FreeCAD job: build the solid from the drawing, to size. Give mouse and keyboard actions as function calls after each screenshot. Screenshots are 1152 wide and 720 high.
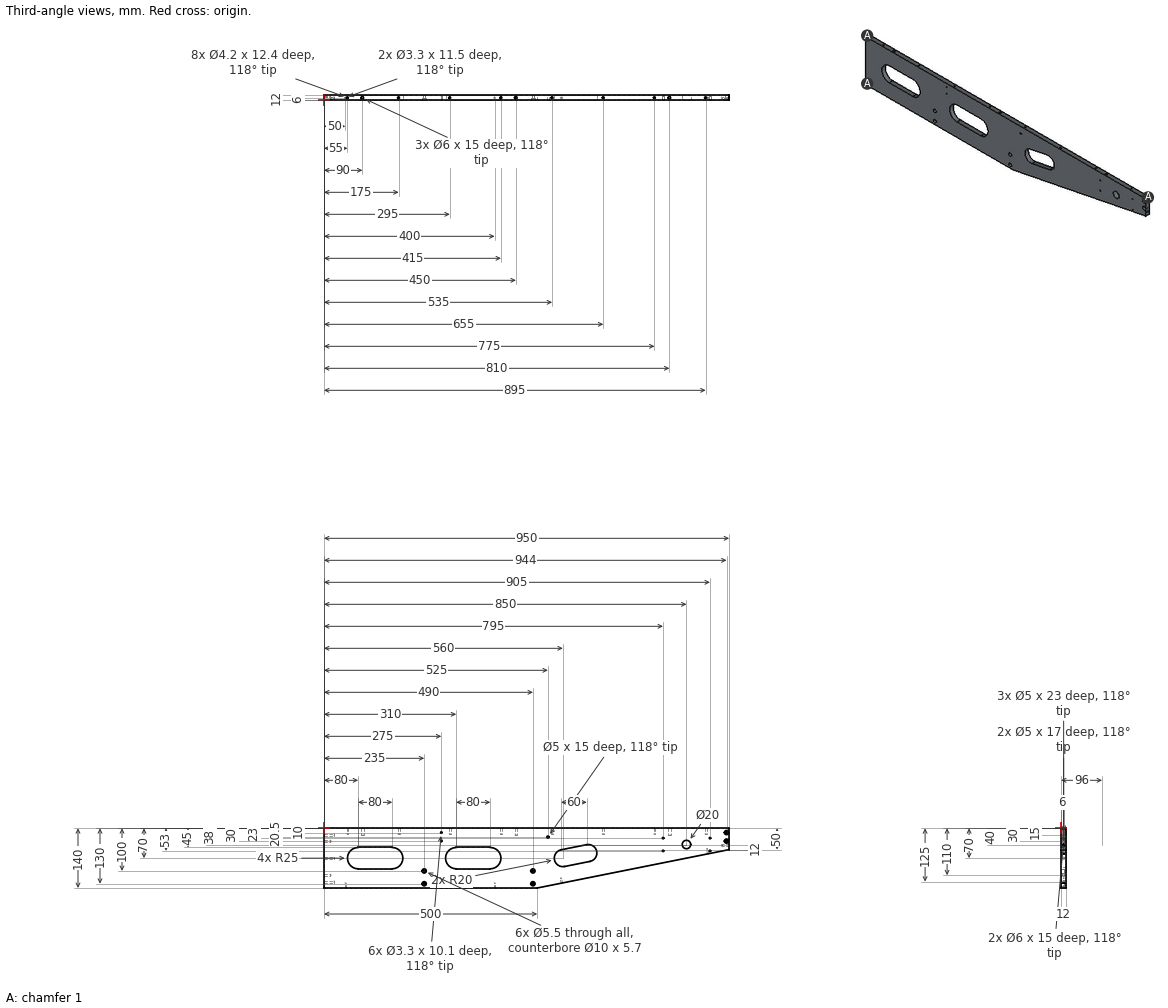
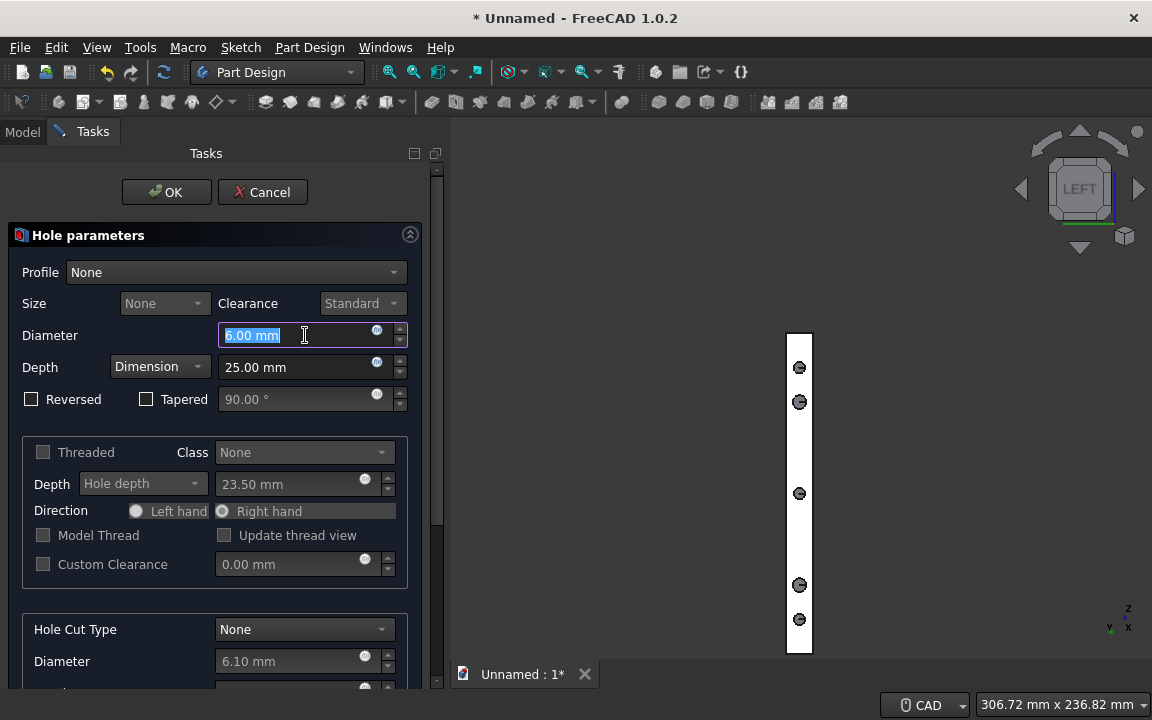
text(4.2)
key(Tab)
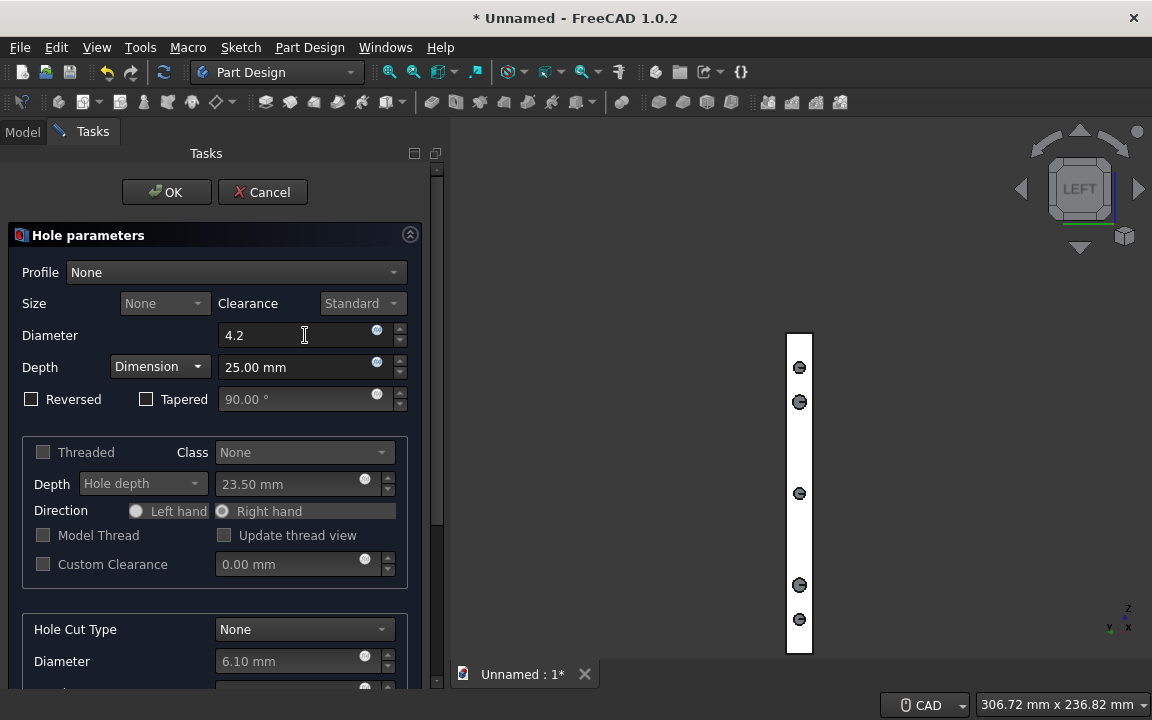
triple_click(305, 367)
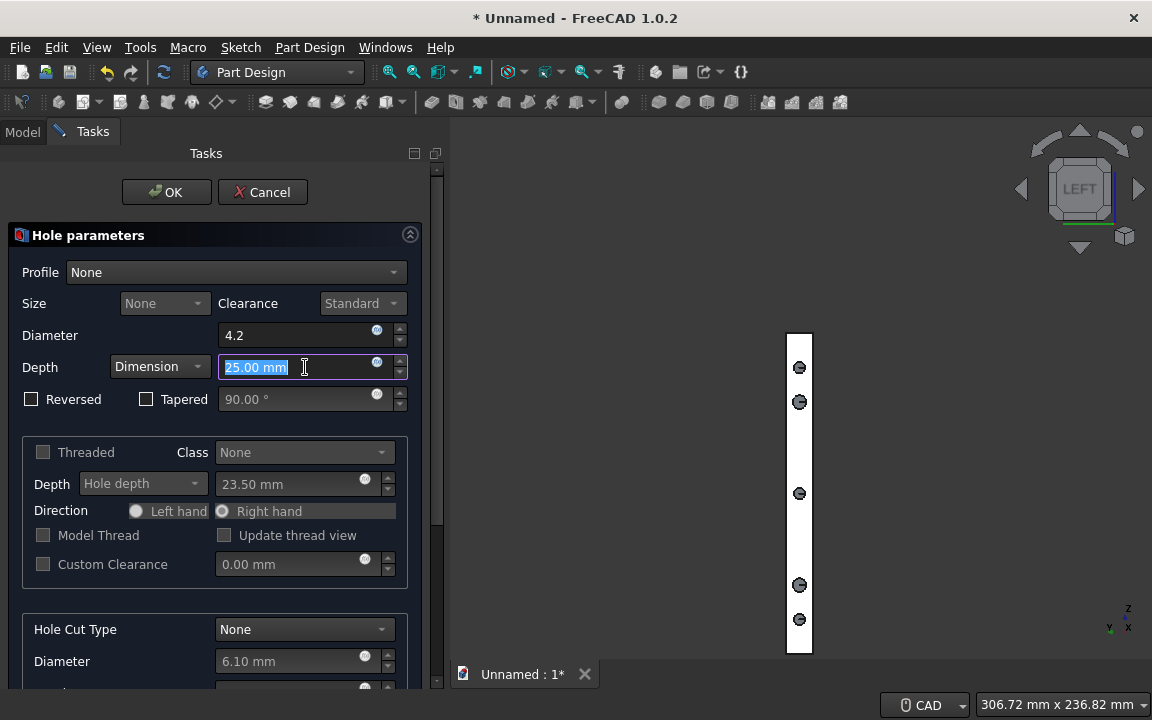
text(12.4)
key(Tab)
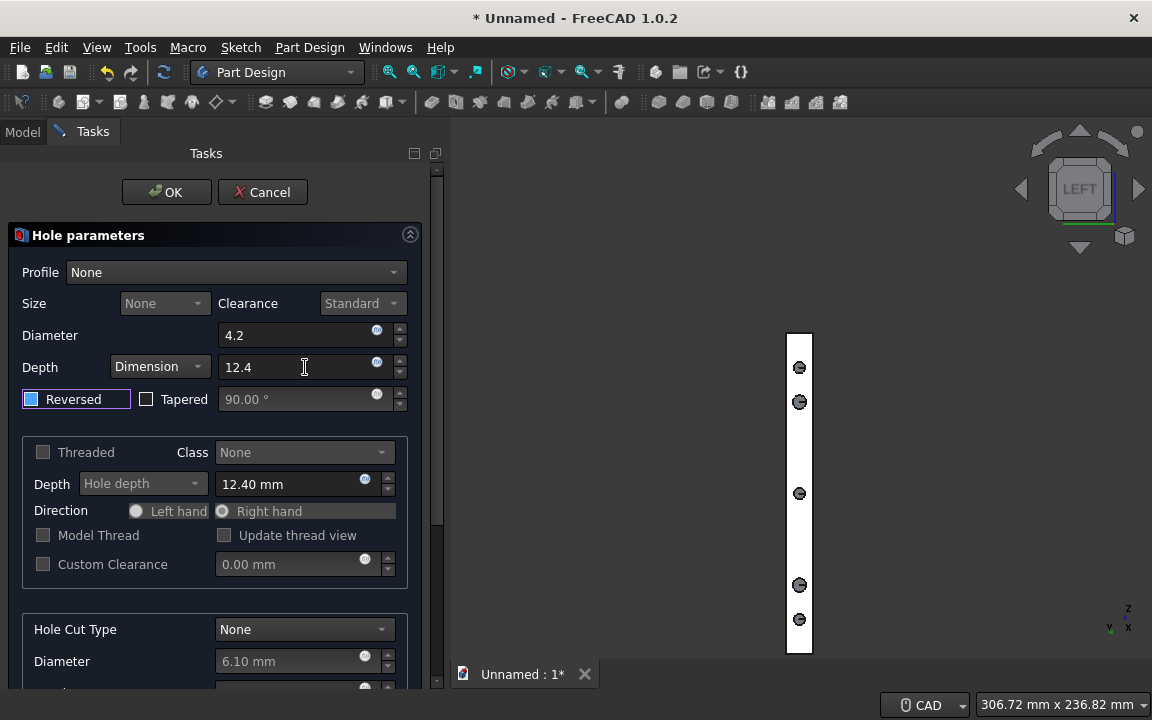
click(167, 192)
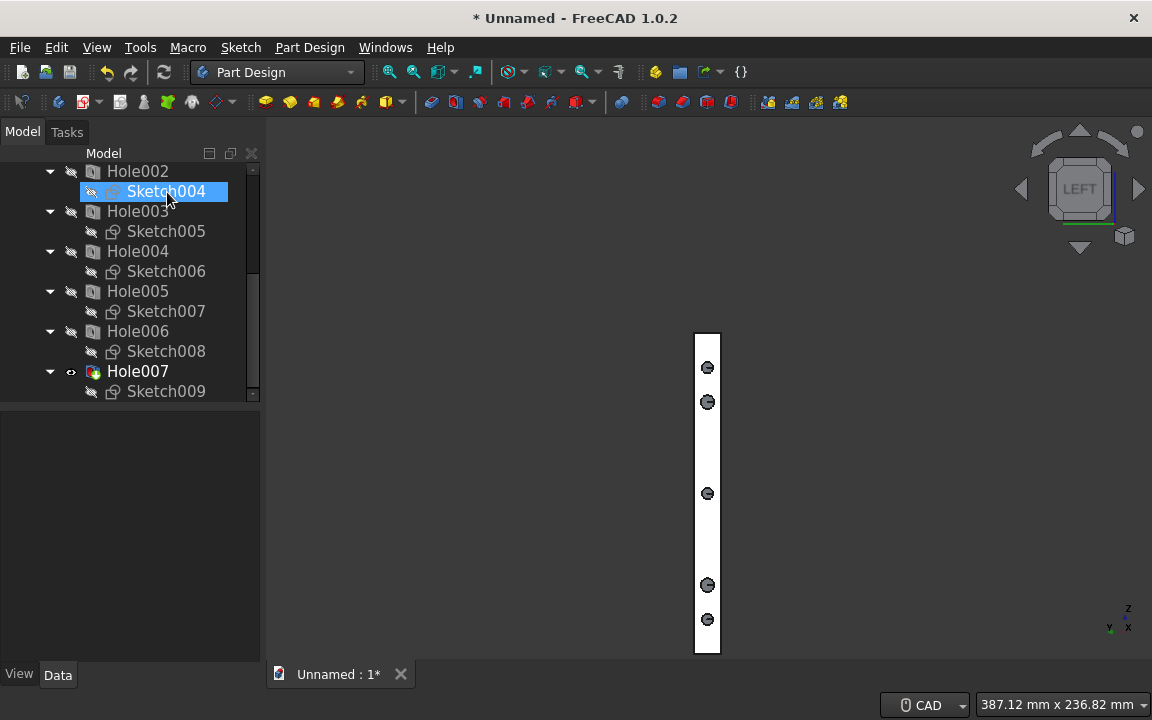
key(0)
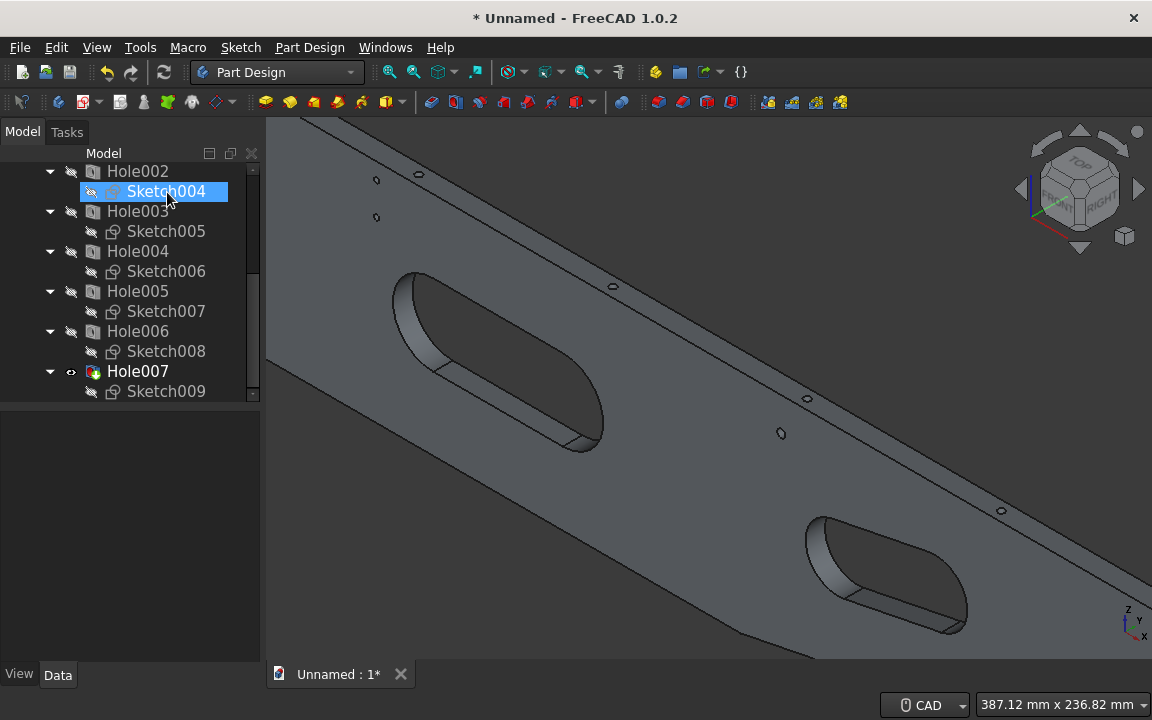
key(v)
key(f)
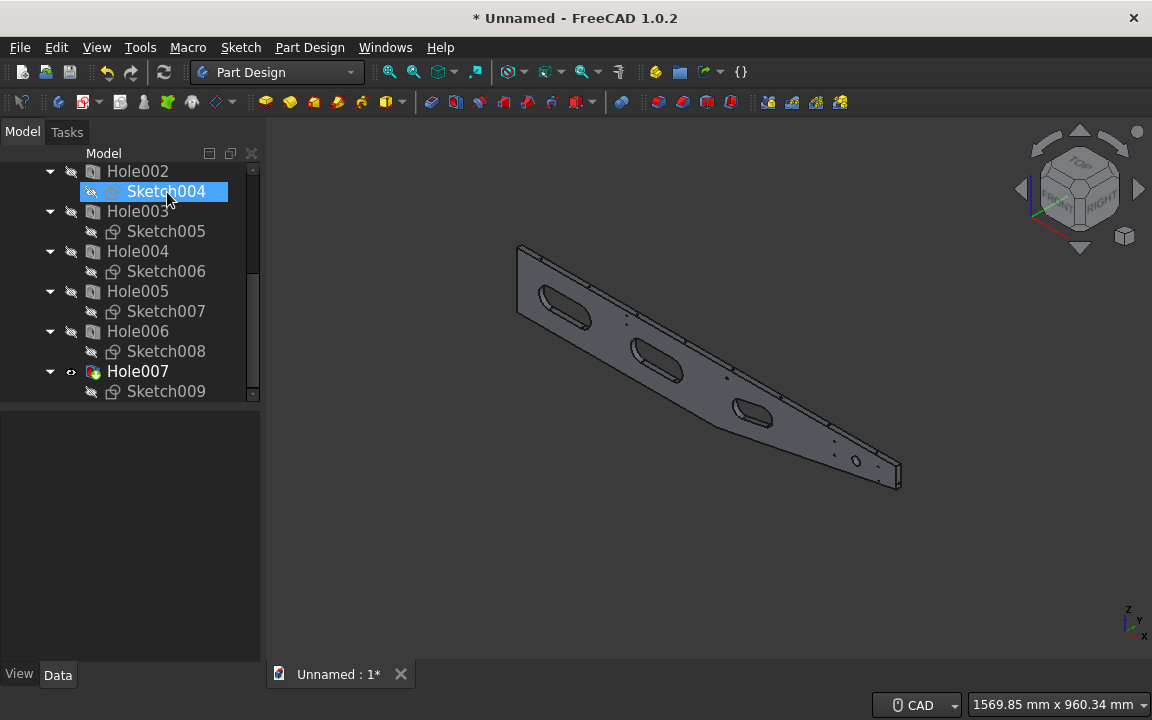
scroll(871, 449, up, 7)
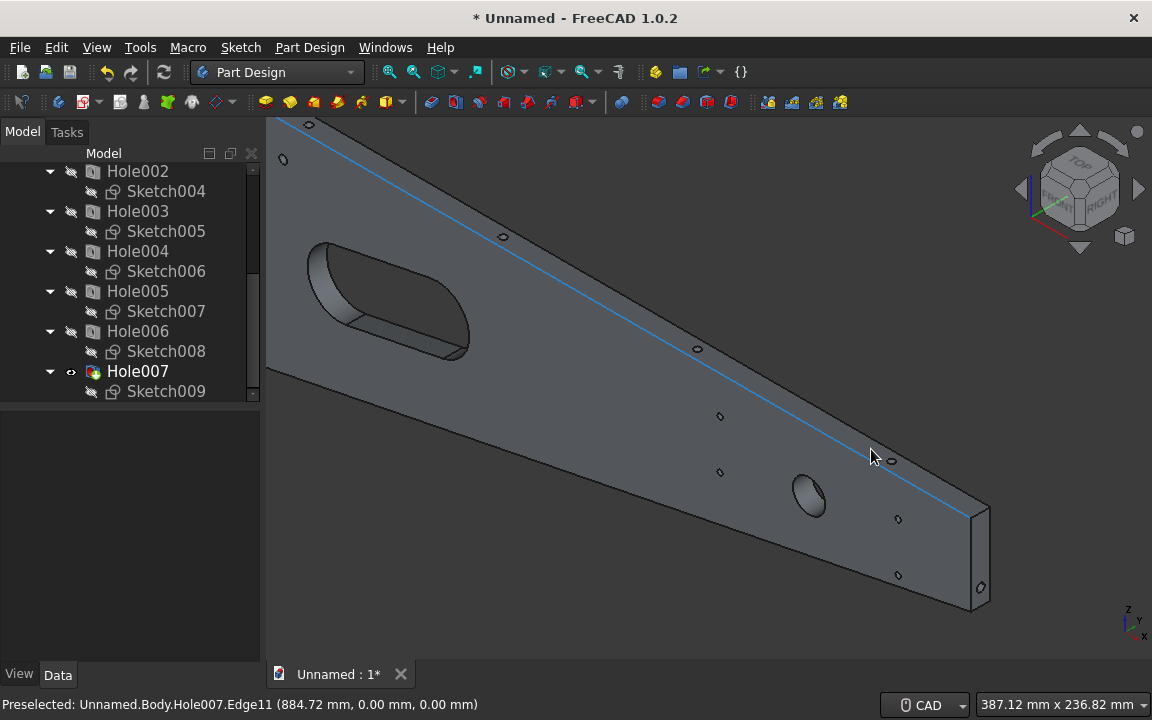
click(871, 448)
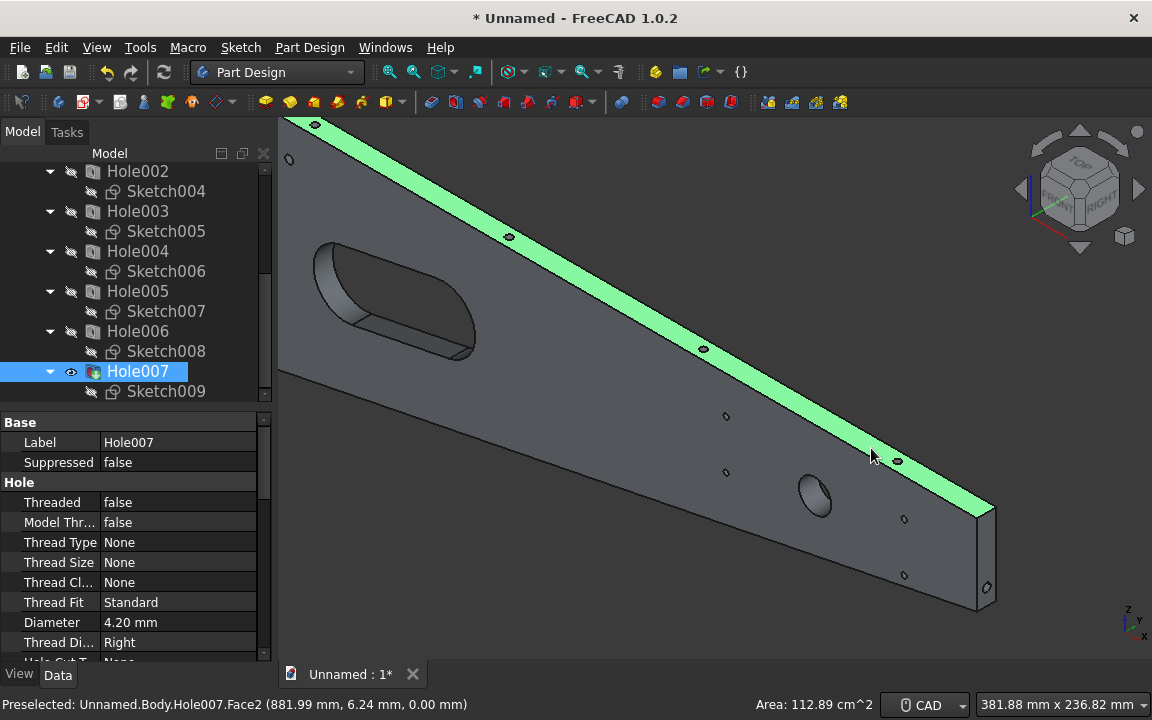
click(84, 102)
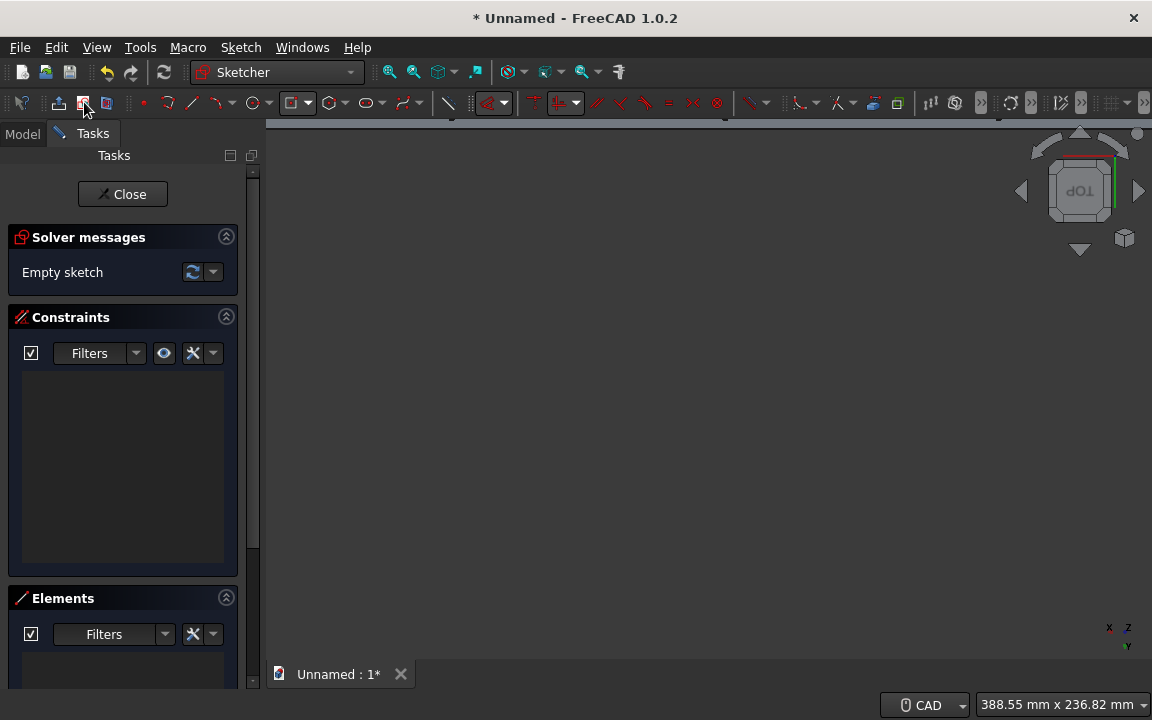
scroll(427, 480, down, 7)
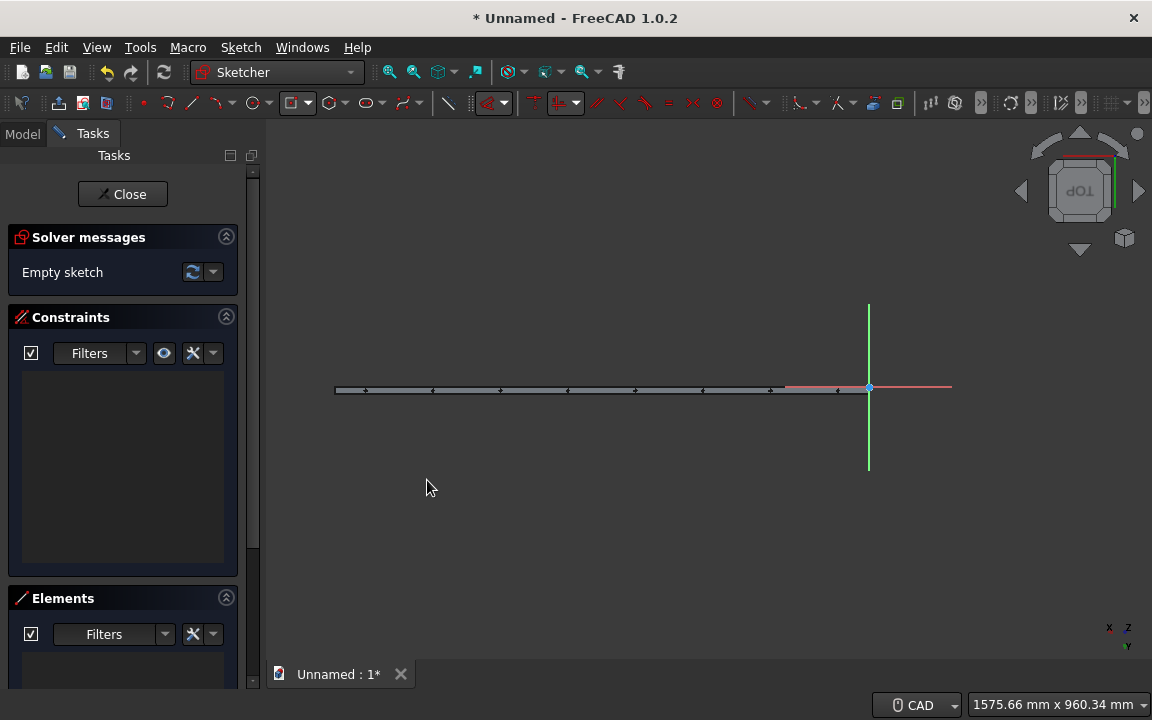
click(254, 104)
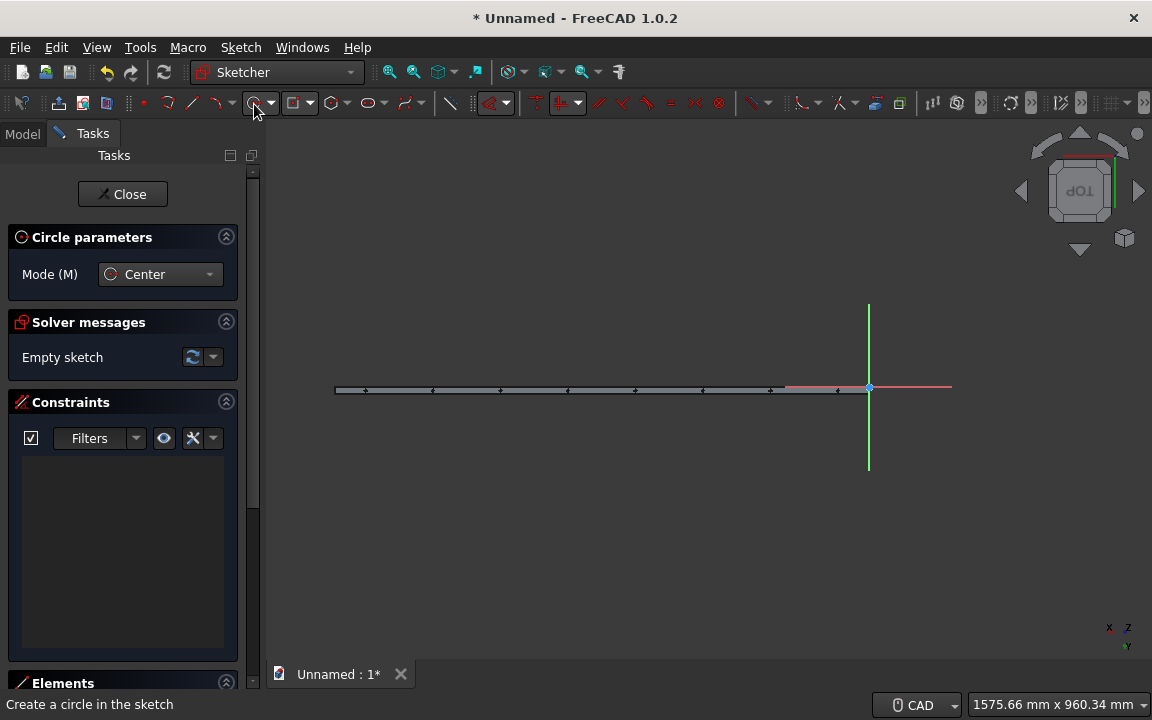
scroll(818, 391, up, 13)